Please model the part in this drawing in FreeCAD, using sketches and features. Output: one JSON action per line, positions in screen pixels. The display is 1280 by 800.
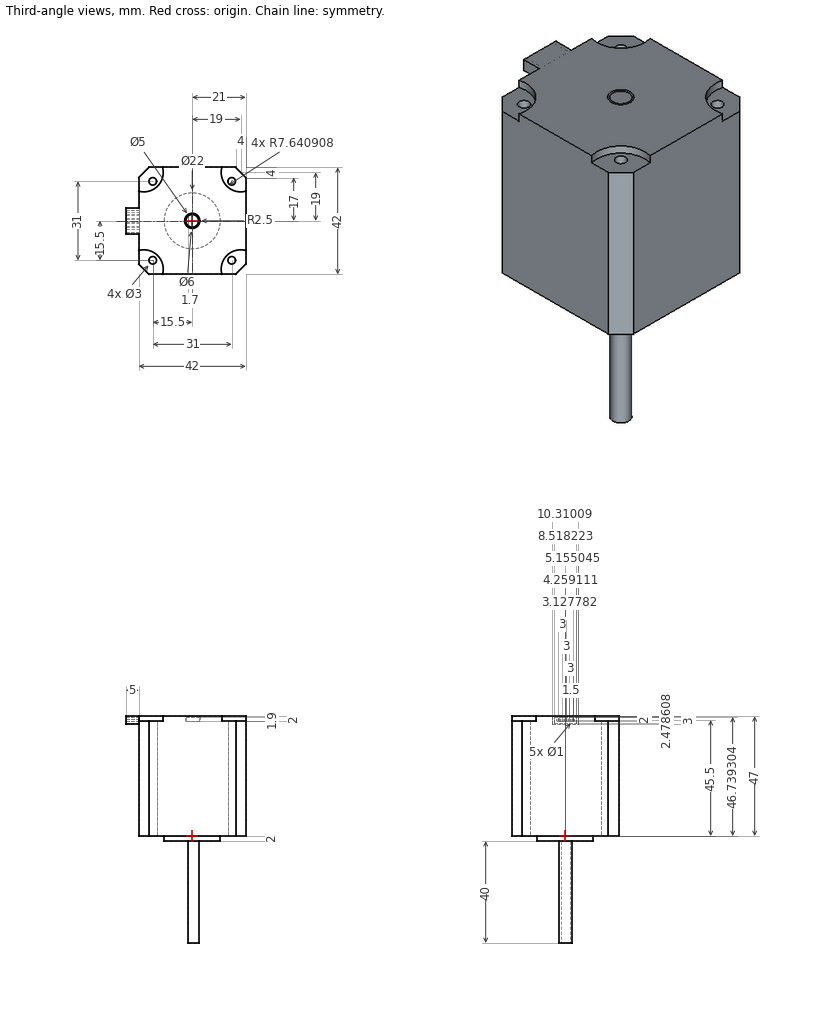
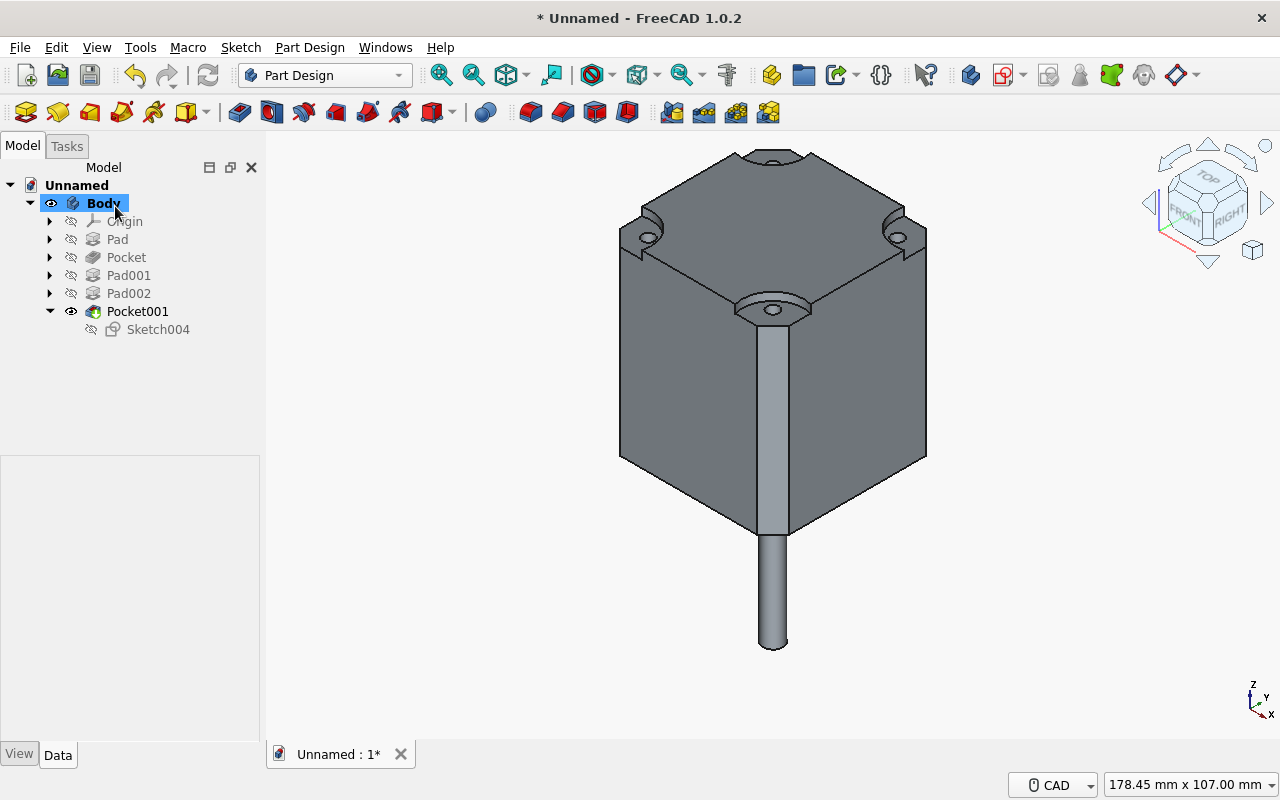
{"action": "left_click", "coordinate": [442, 76]}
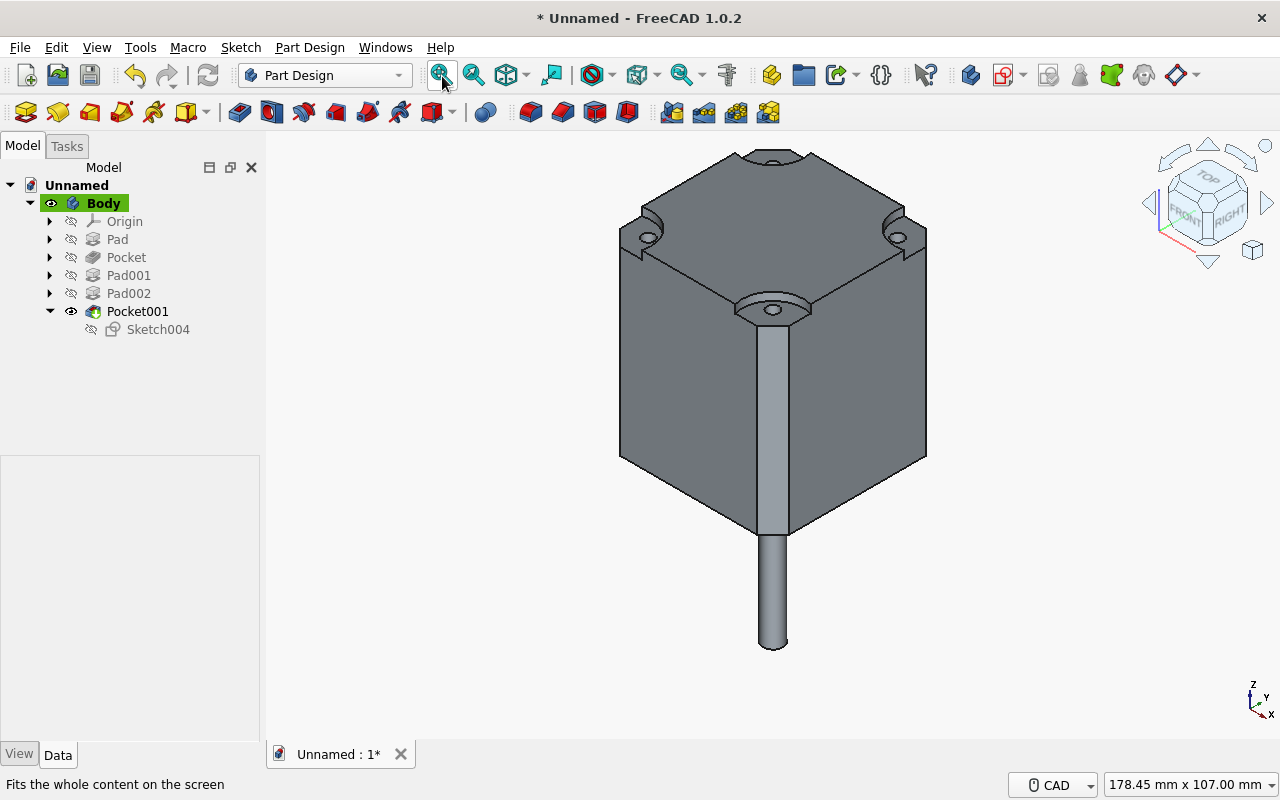
{"action": "left_click", "coordinate": [773, 228]}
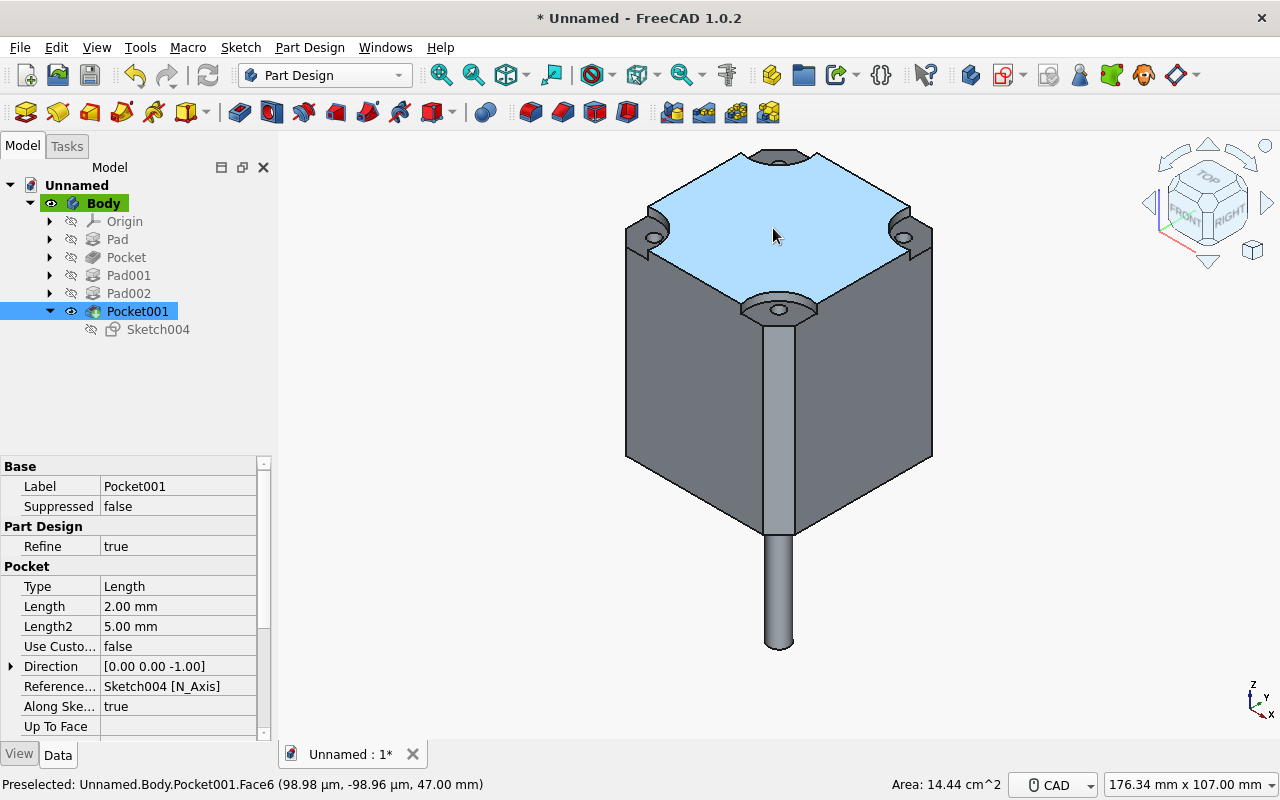
{"action": "left_click", "coordinate": [1004, 76]}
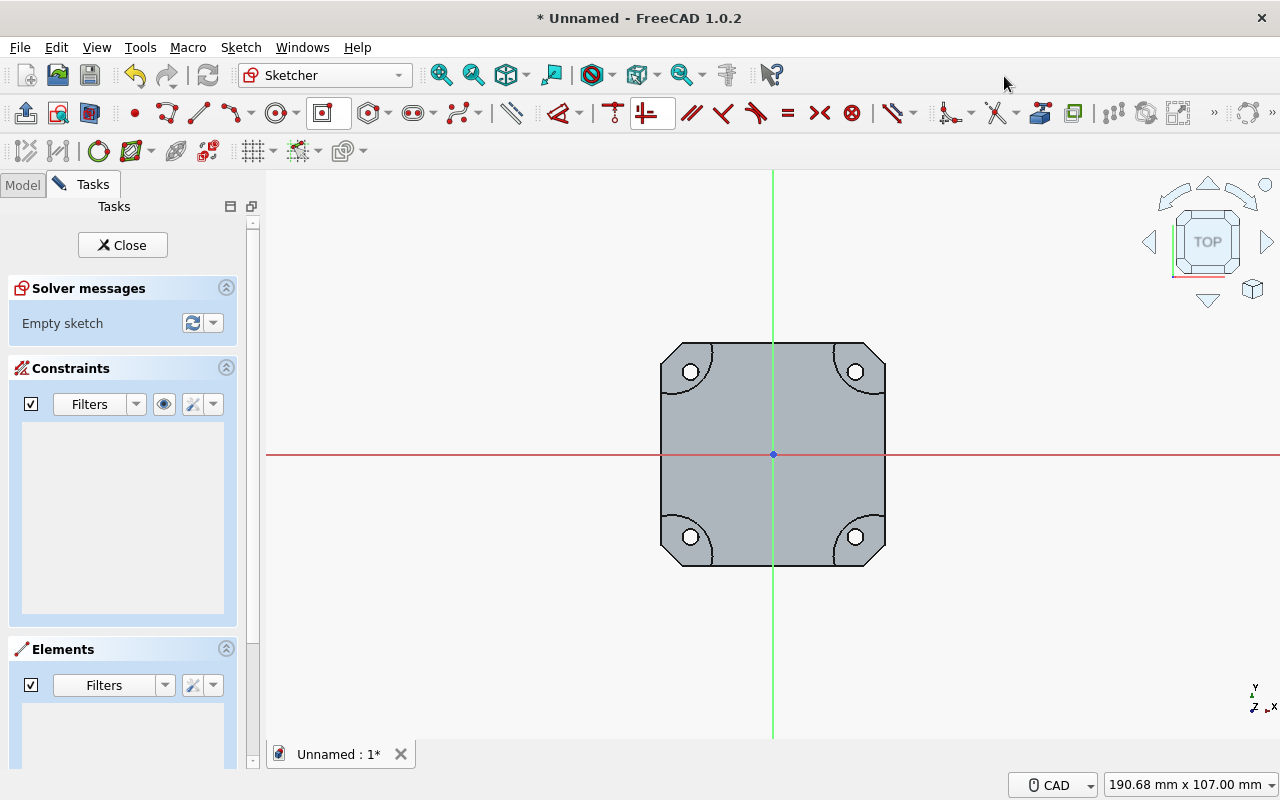
{"action": "scroll", "coordinate": [780, 455], "scroll_direction": "up", "scroll_amount": 12}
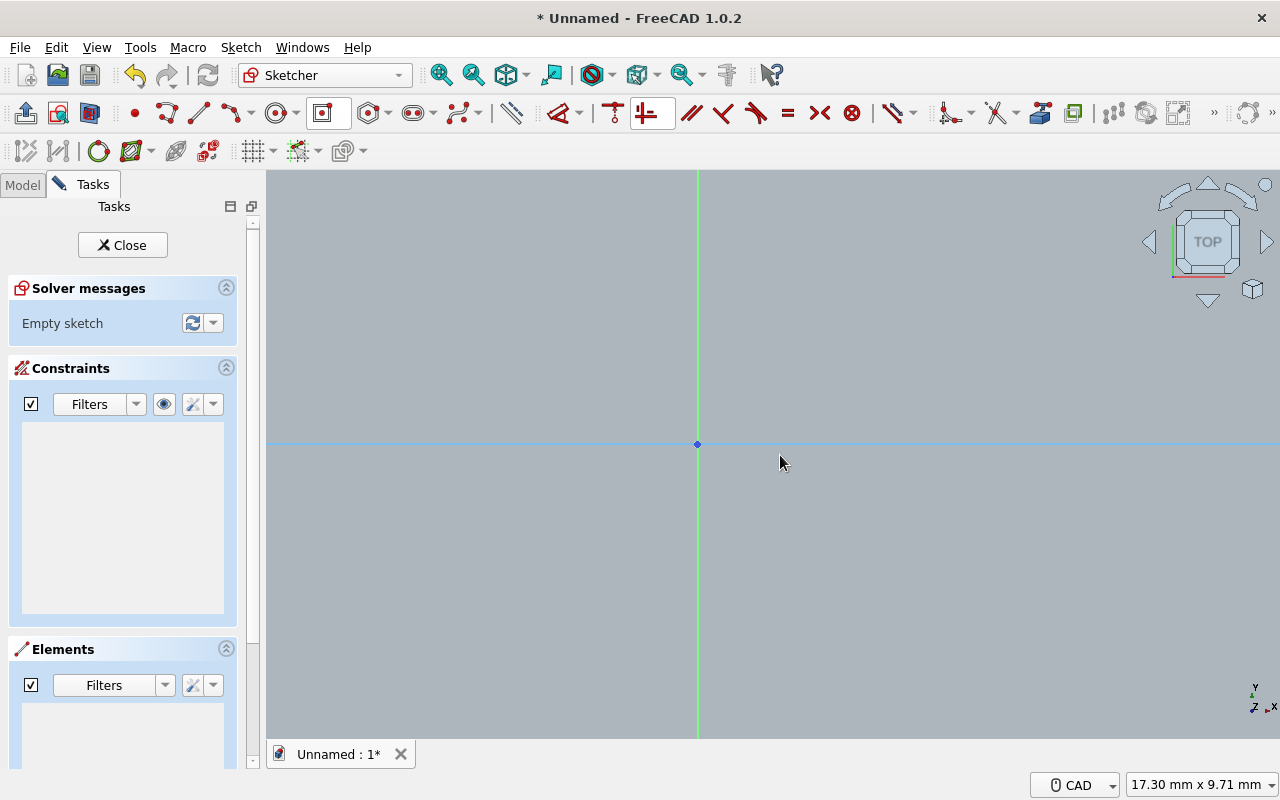
{"action": "left_click", "coordinate": [276, 114]}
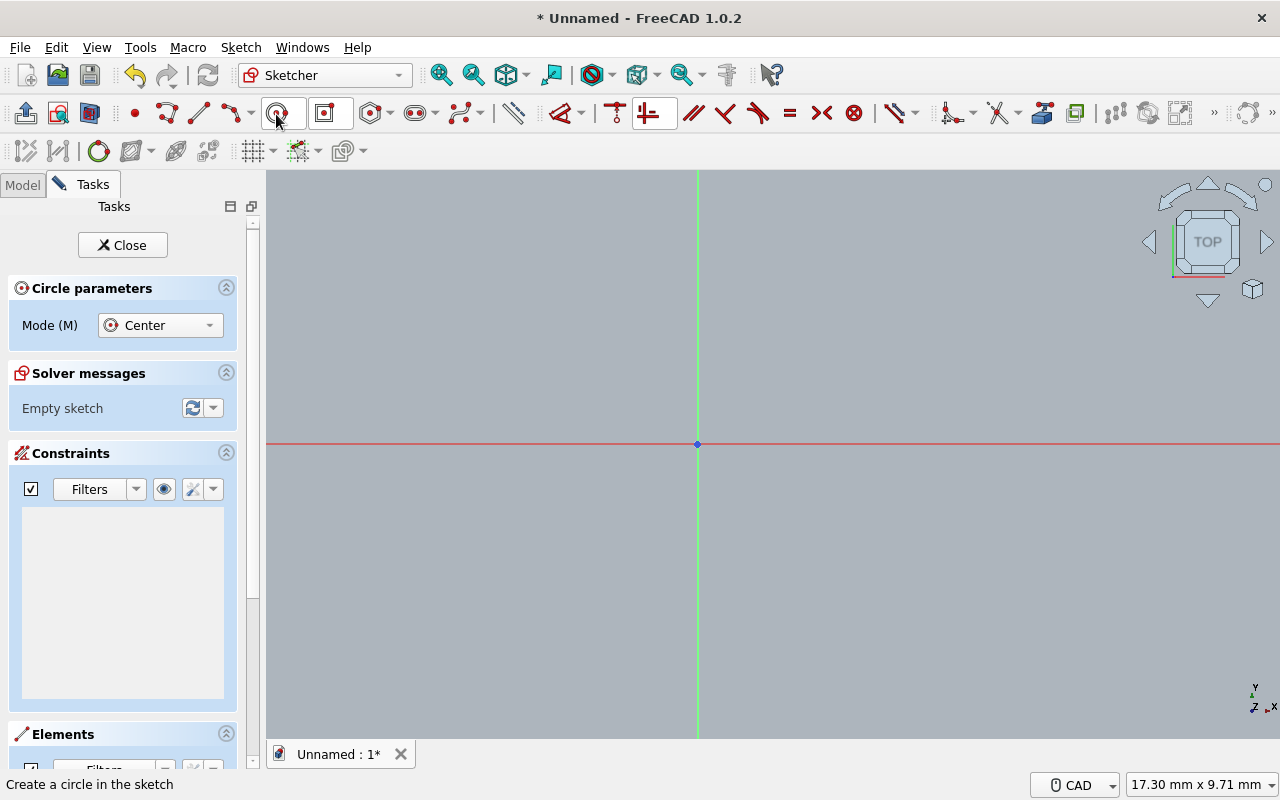
{"action": "left_click", "coordinate": [698, 444]}
{"action": "left_click", "coordinate": [822, 320]}
{"action": "key", "text": "Escape"}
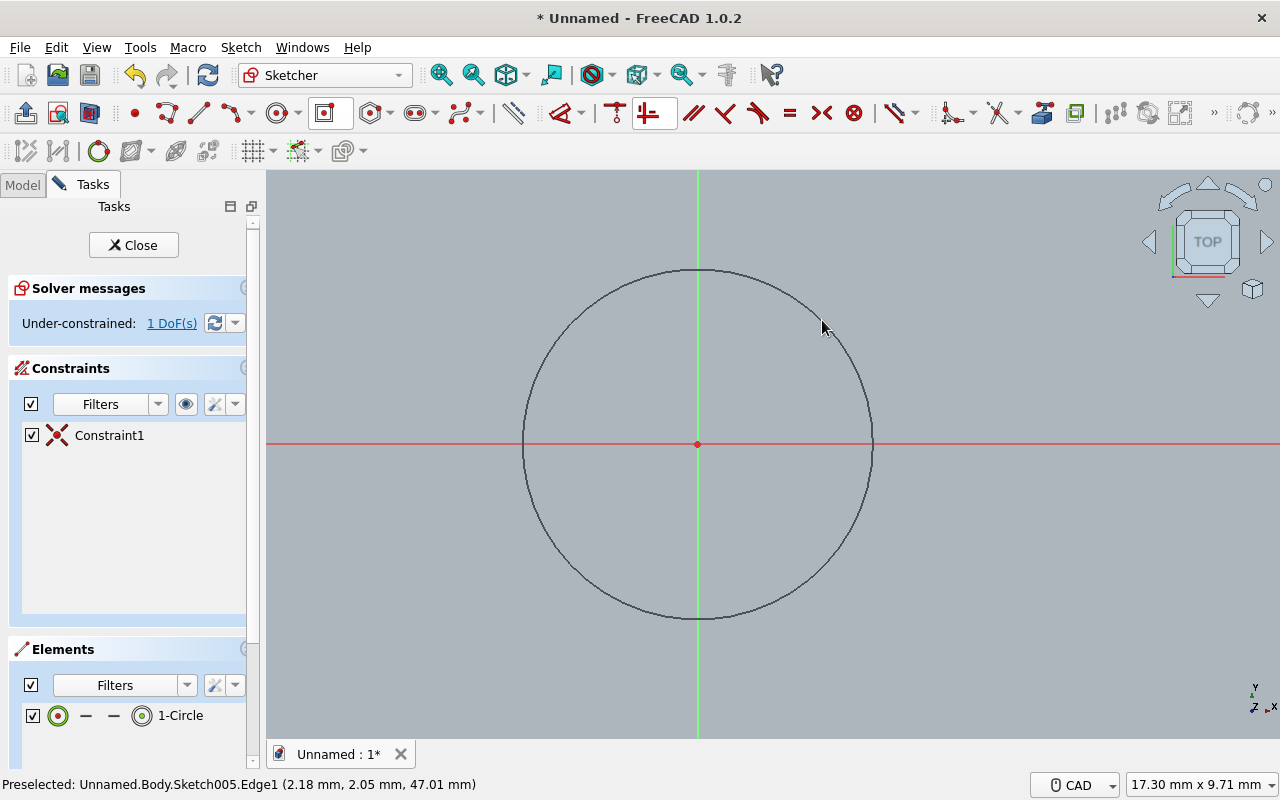
{"action": "key", "text": "d"}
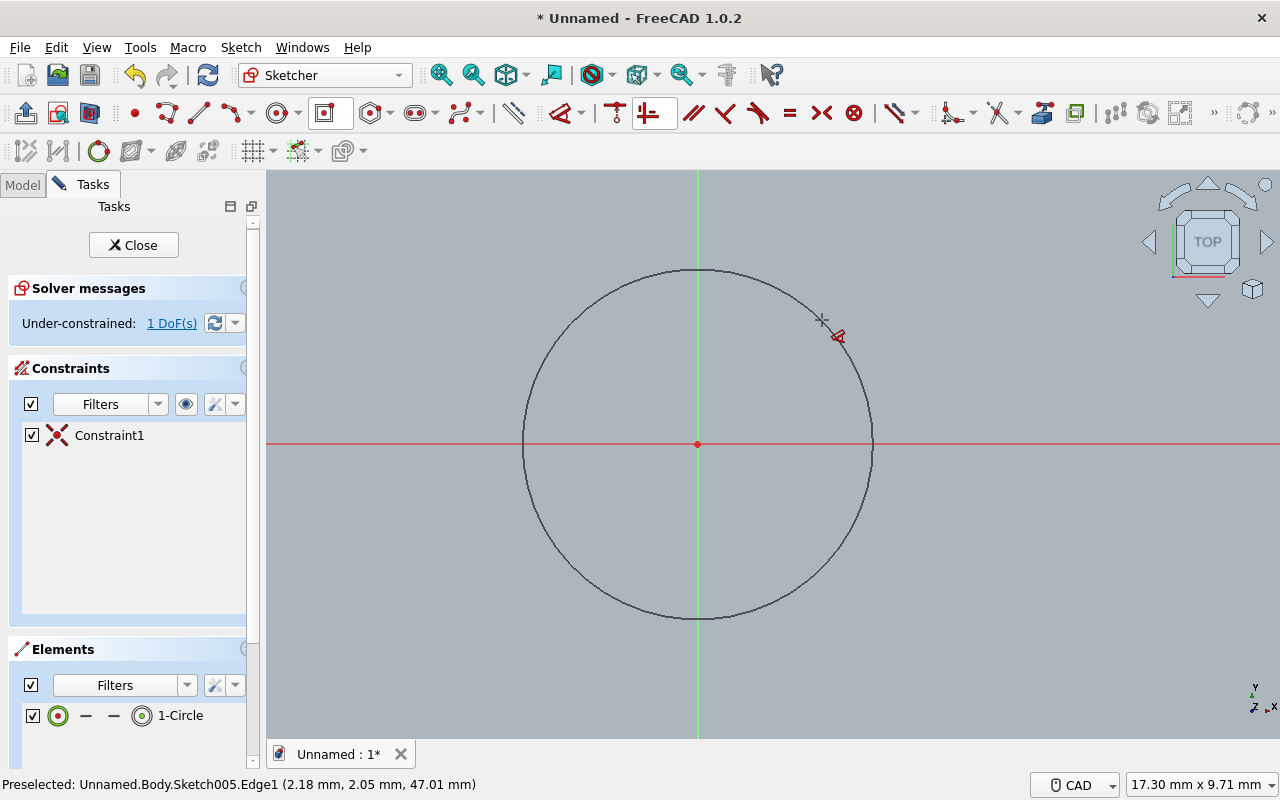
{"action": "left_click", "coordinate": [821, 320]}
{"action": "left_click", "coordinate": [844, 297]}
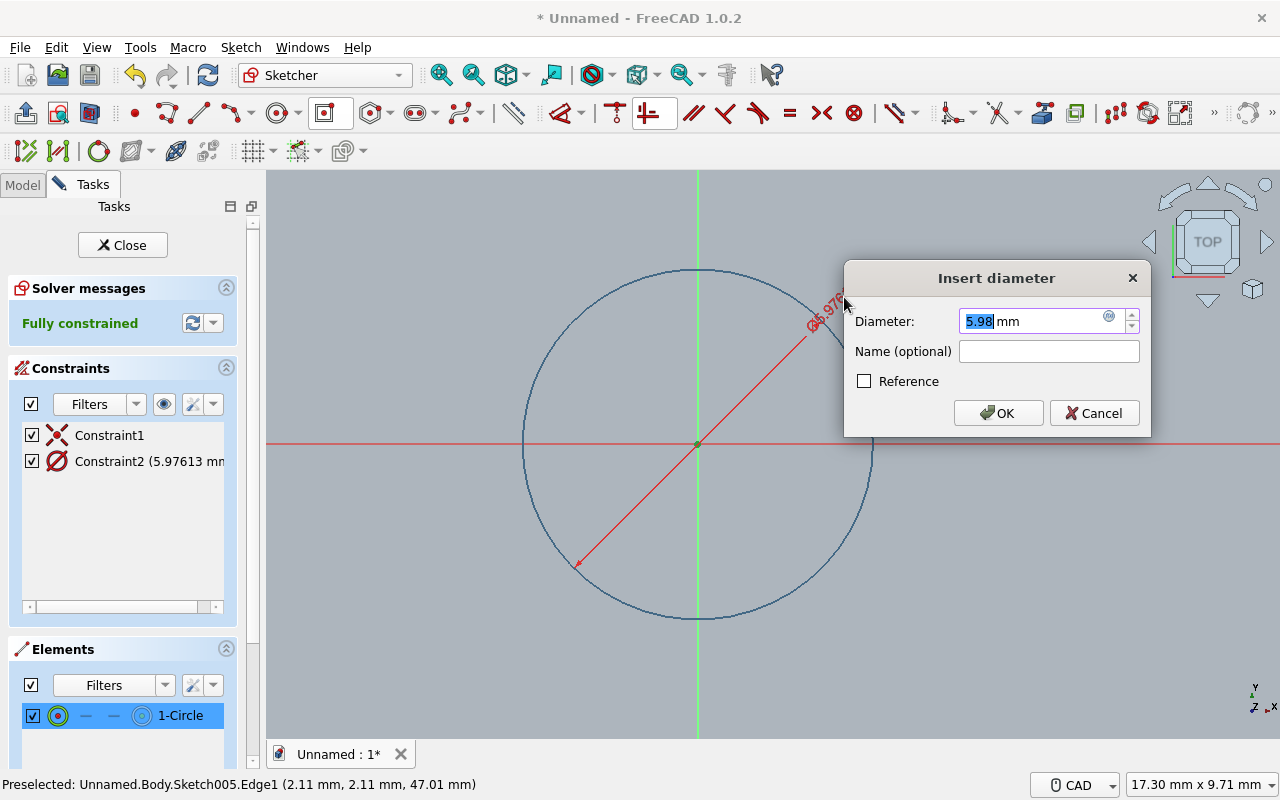
{"action": "type", "text": "6"}
{"action": "key", "text": "Return"}
{"action": "key", "text": "Escape"}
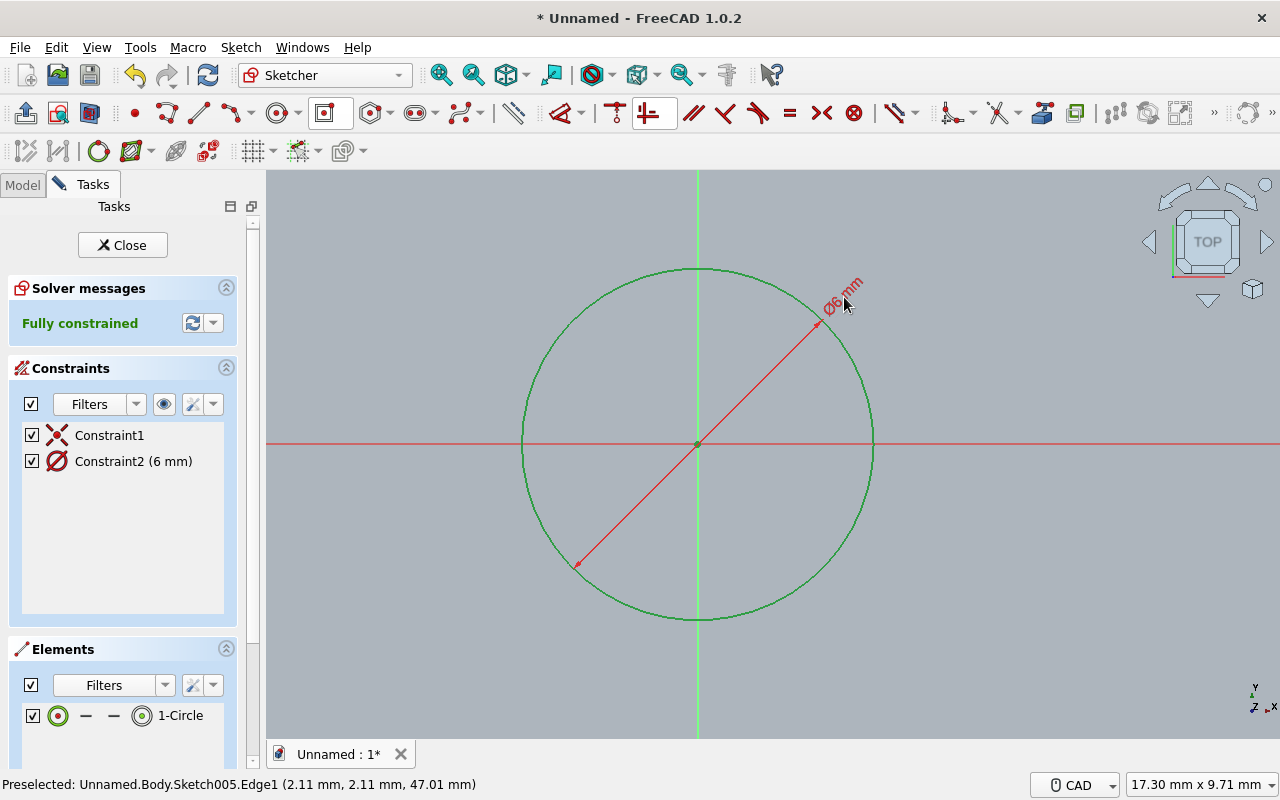
{"action": "left_click", "coordinate": [123, 245]}